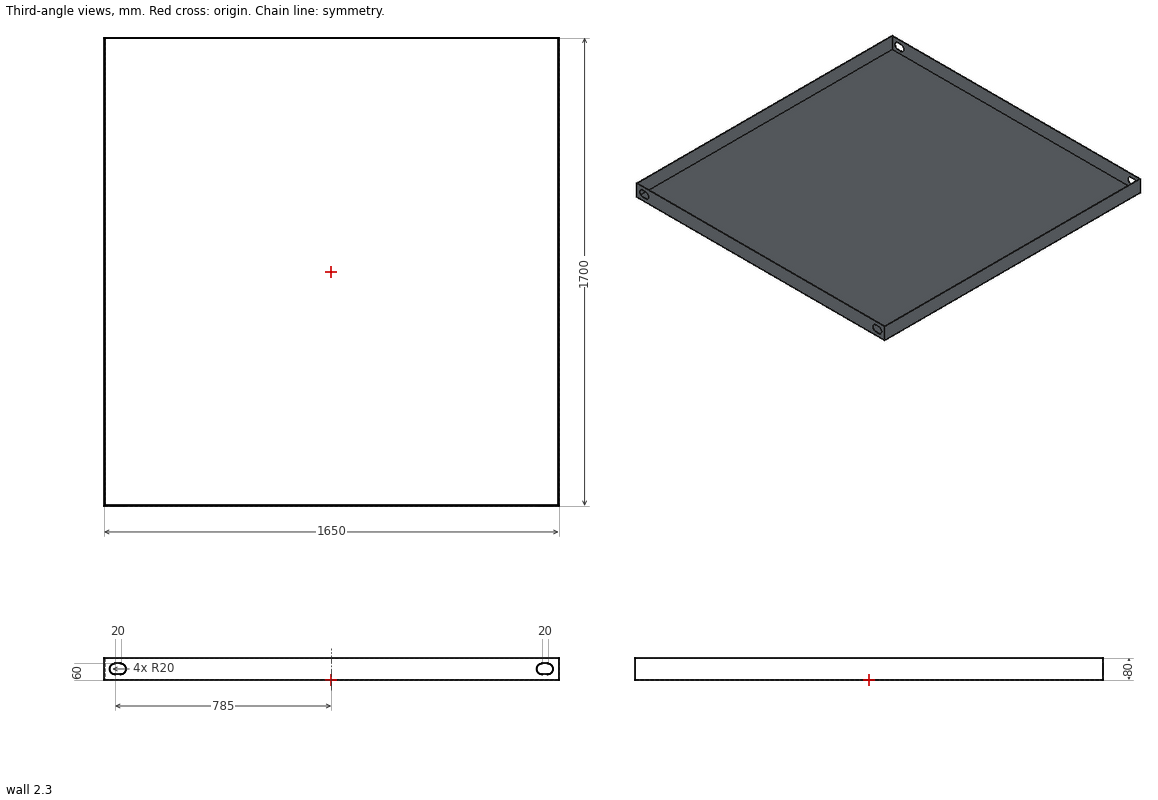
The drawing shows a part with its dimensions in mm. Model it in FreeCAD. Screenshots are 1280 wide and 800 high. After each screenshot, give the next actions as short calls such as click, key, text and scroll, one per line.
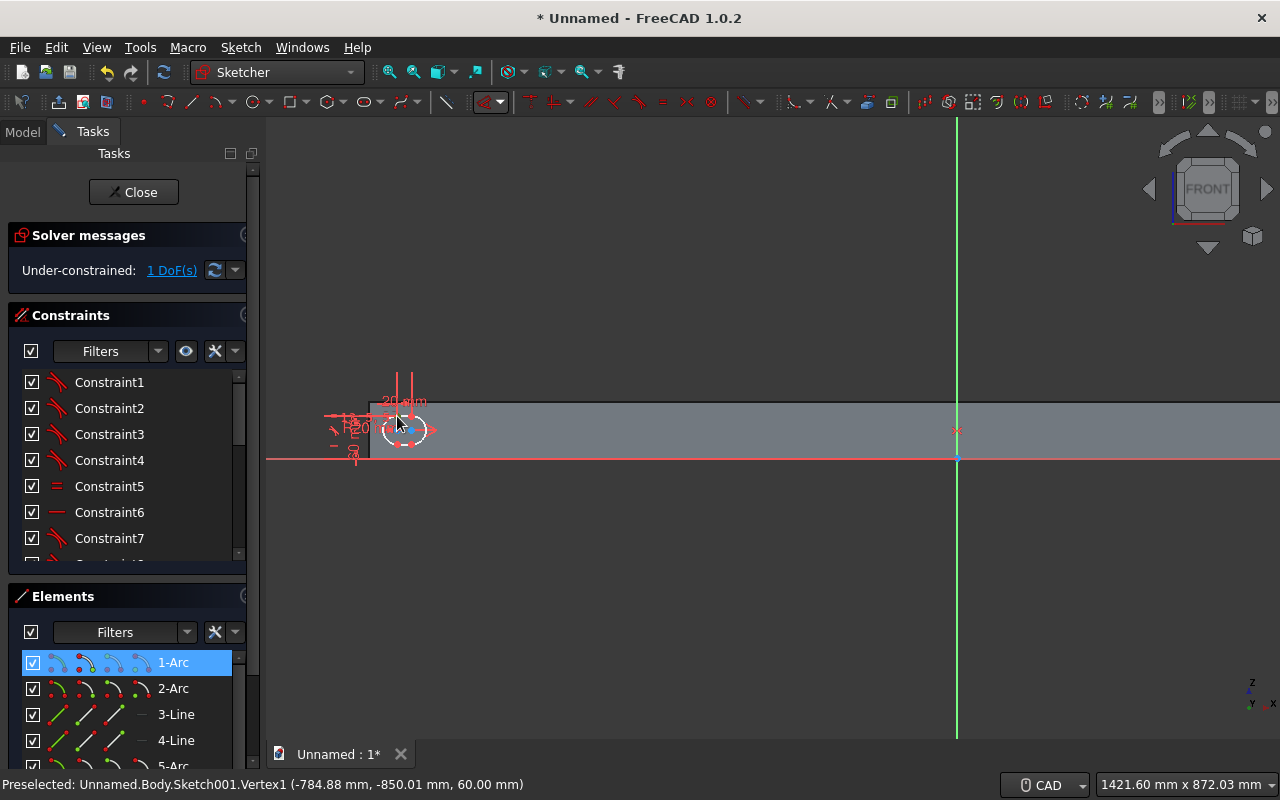
click(502, 102)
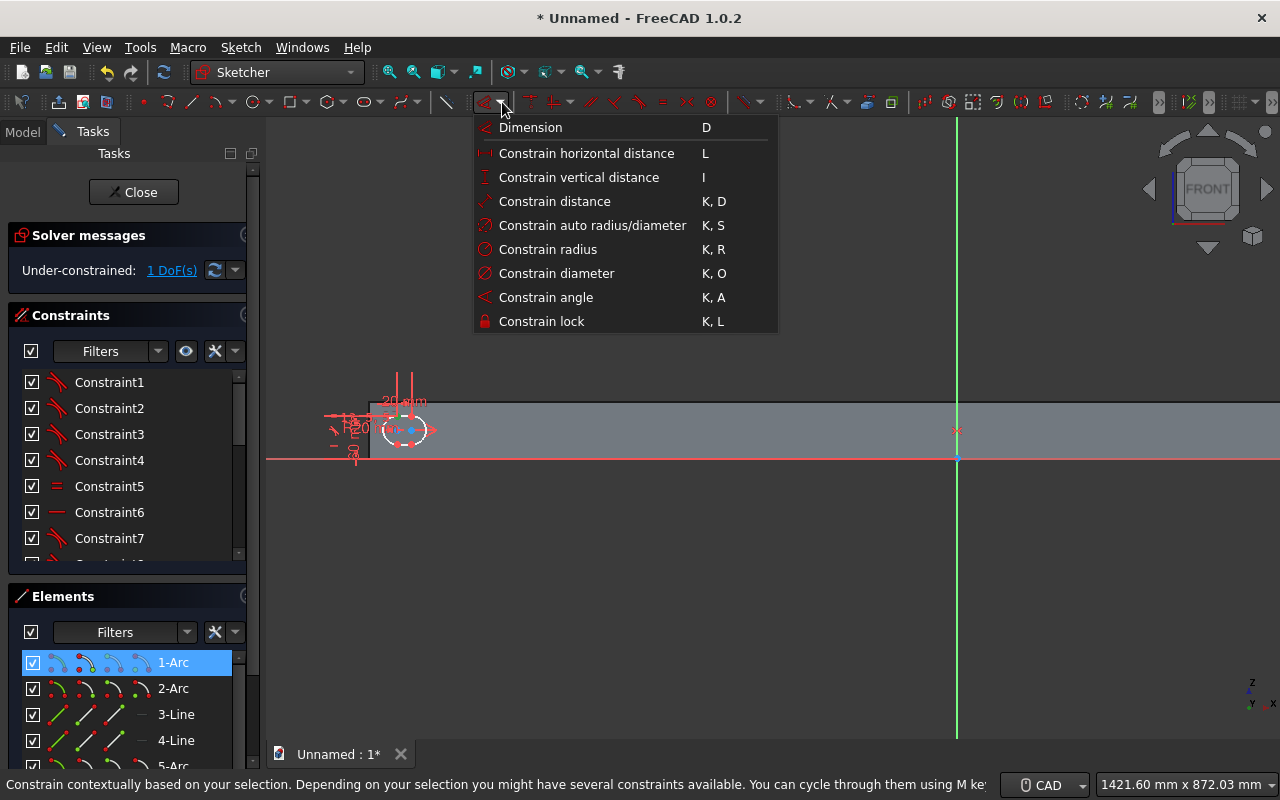
click(626, 153)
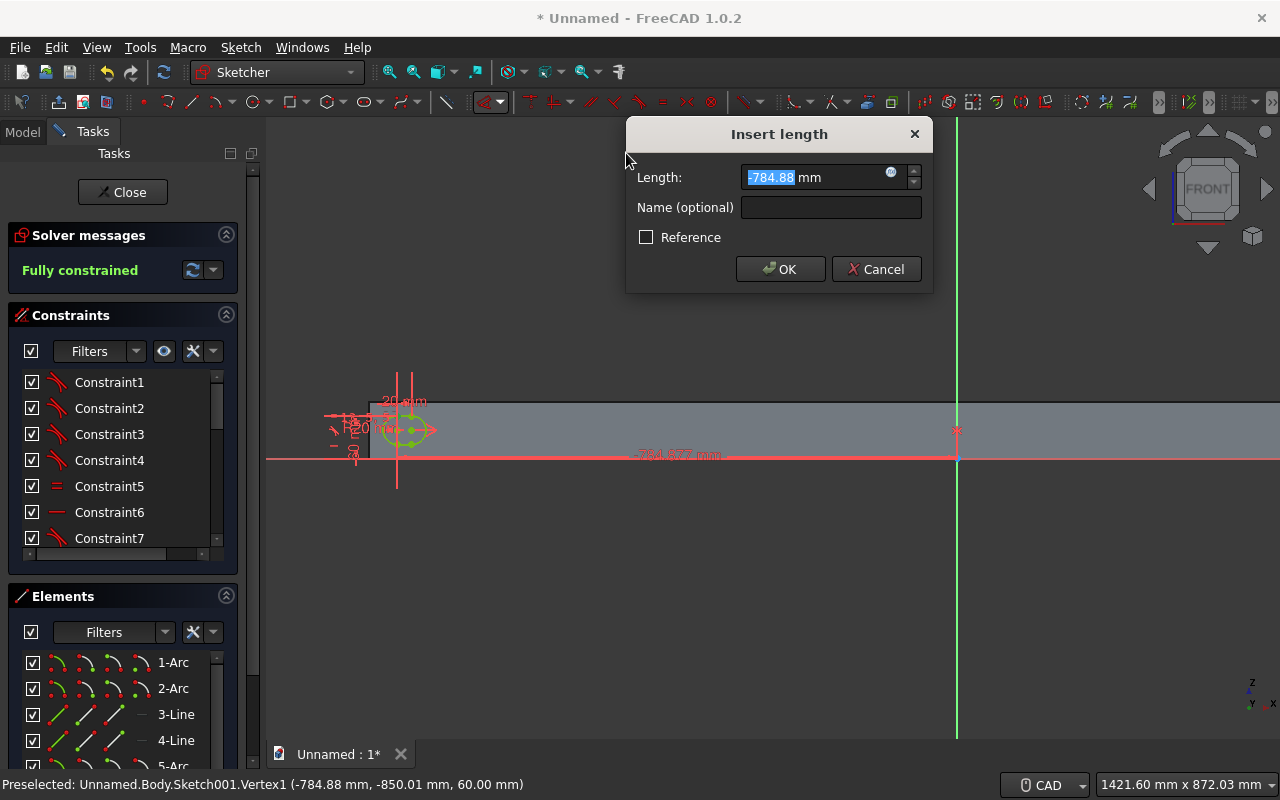
text(-785)
key(Return)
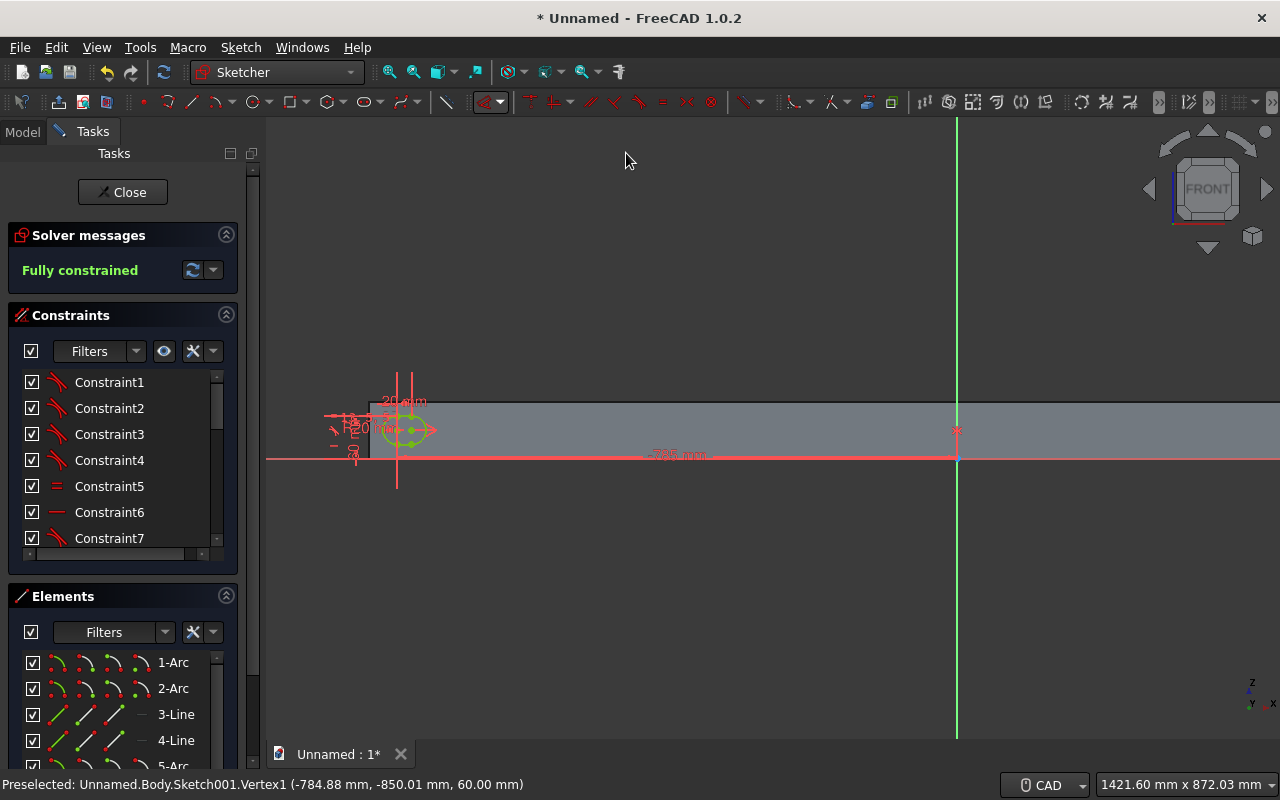
click(123, 192)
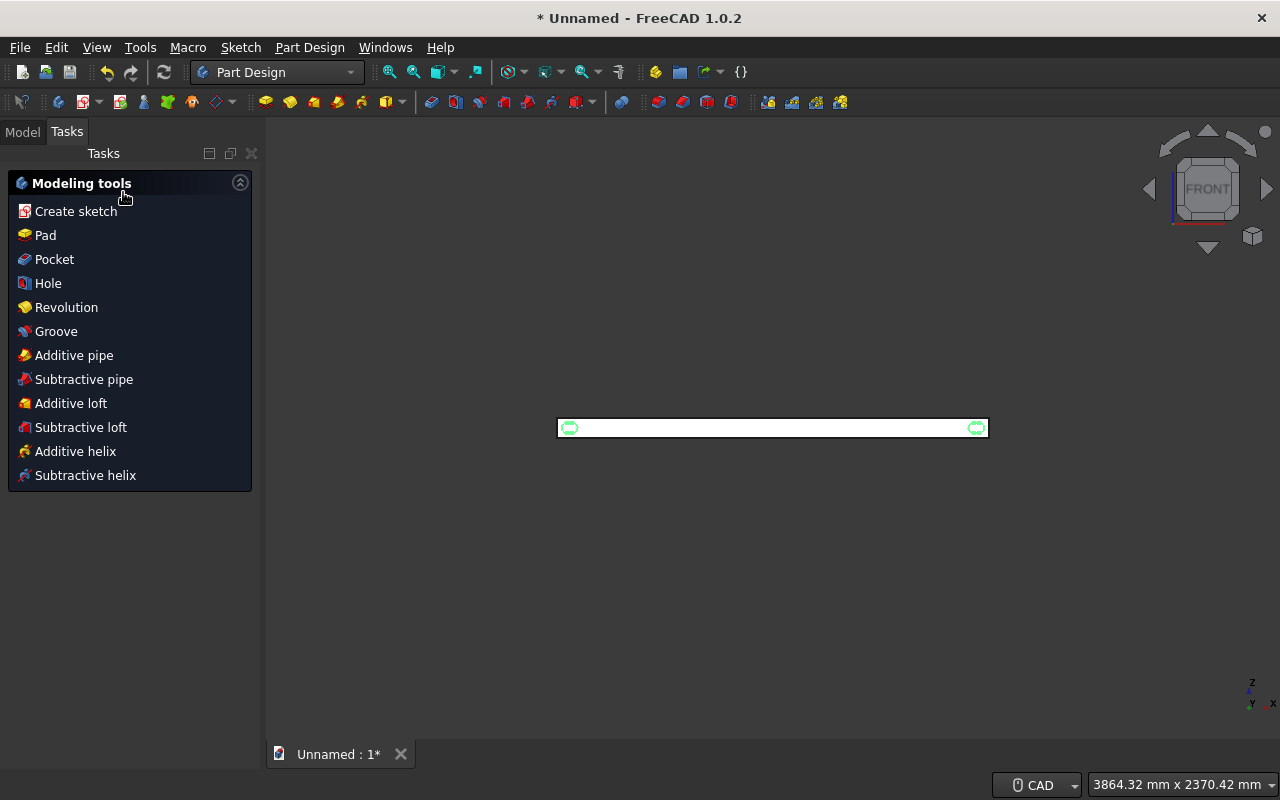
click(432, 102)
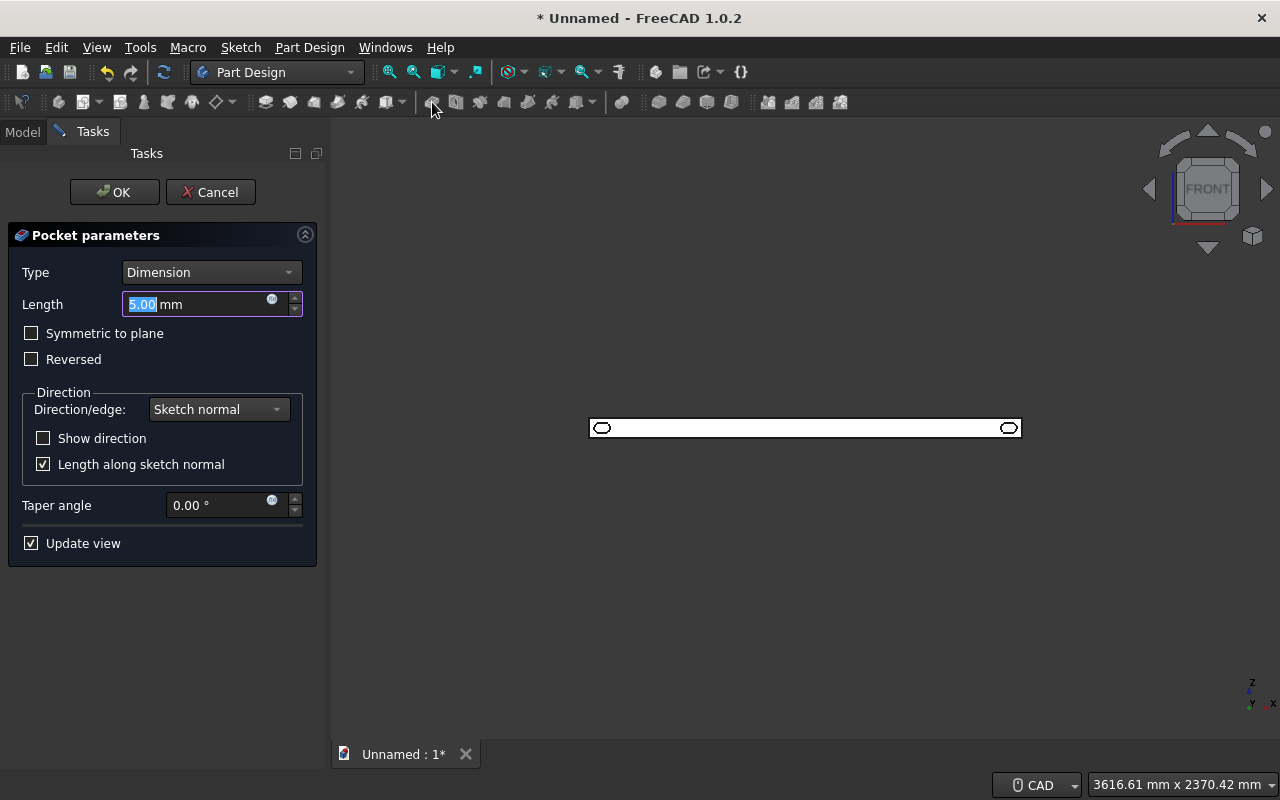
click(212, 272)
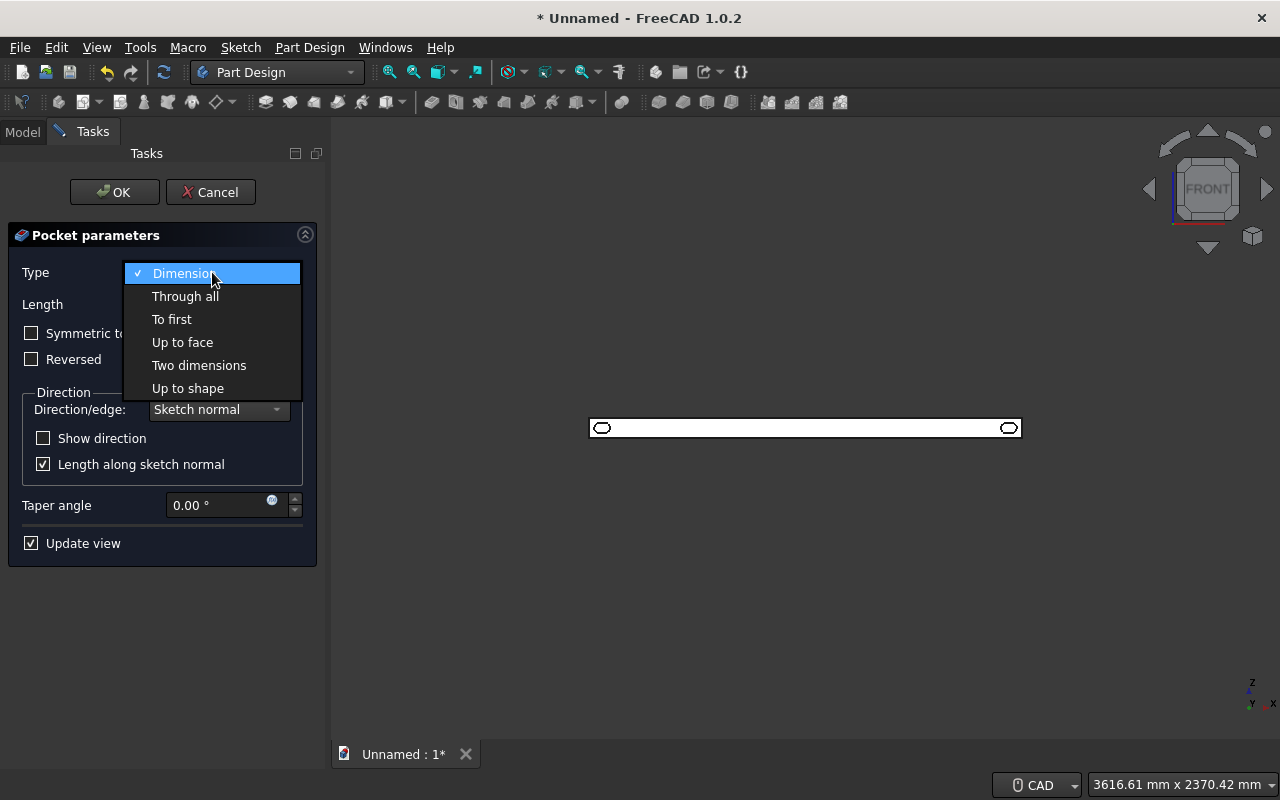
click(212, 296)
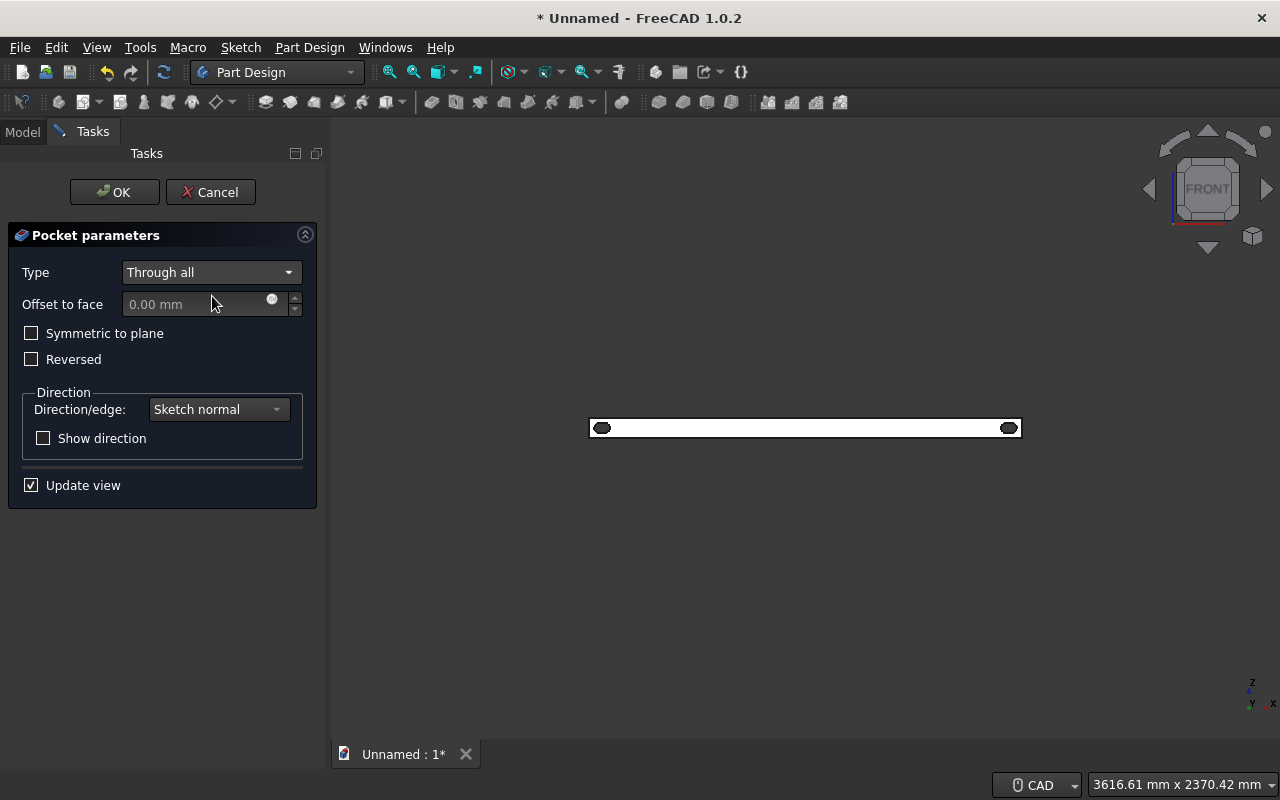
click(115, 192)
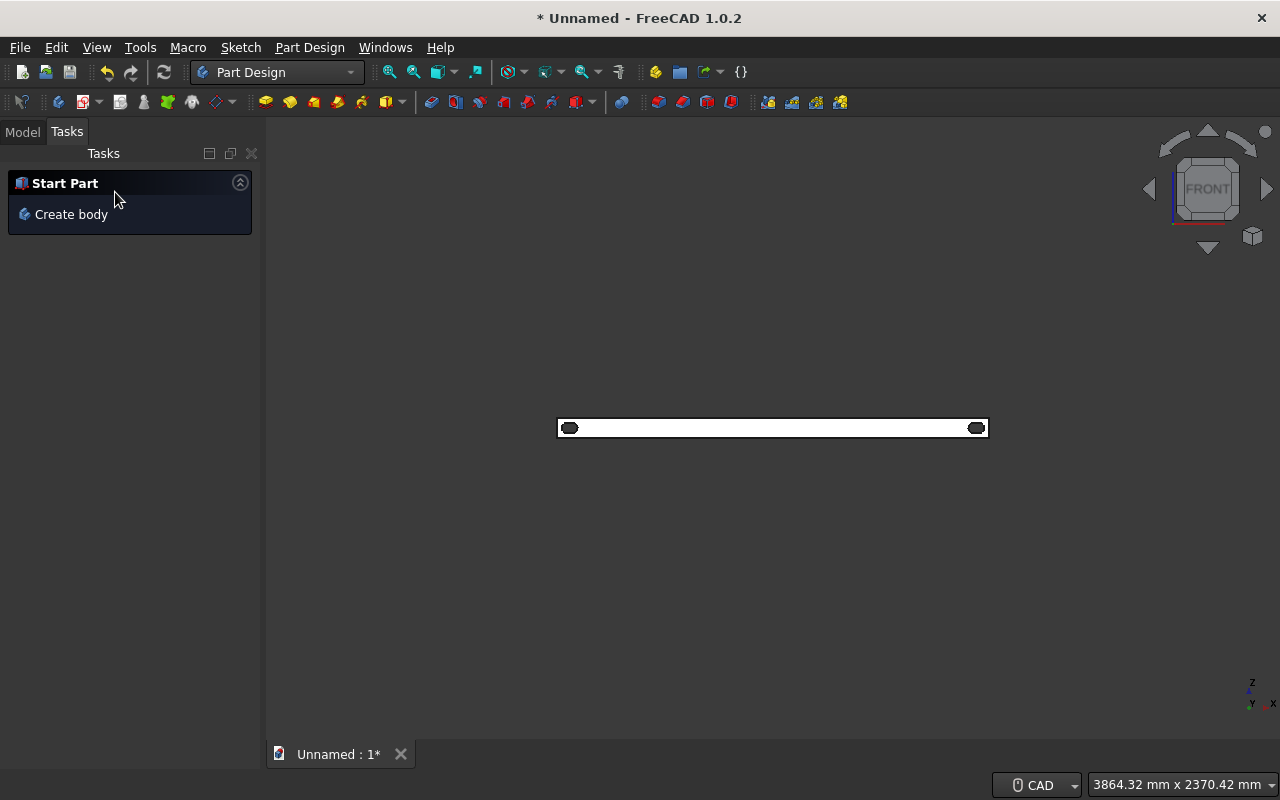
key(0)